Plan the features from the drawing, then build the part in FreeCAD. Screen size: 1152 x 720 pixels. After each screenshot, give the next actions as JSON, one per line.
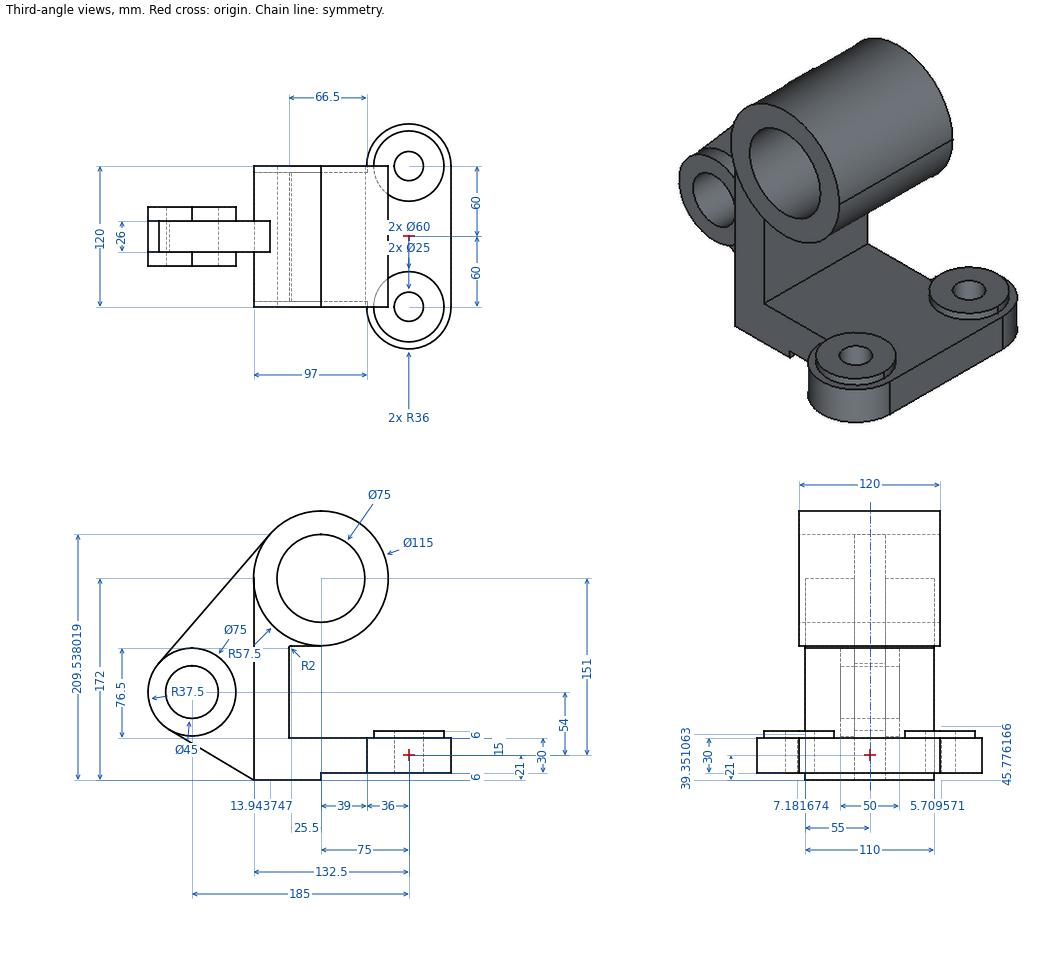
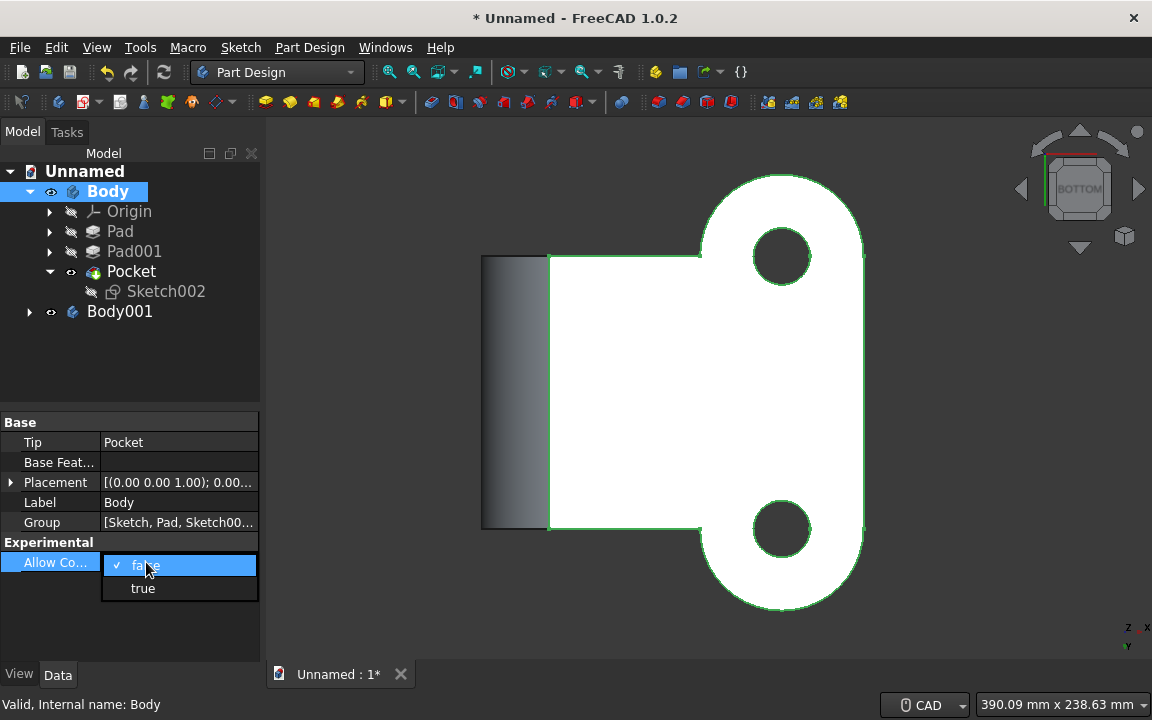
{"action": "left_click", "coordinate": [179, 588]}
{"action": "key", "text": "Return"}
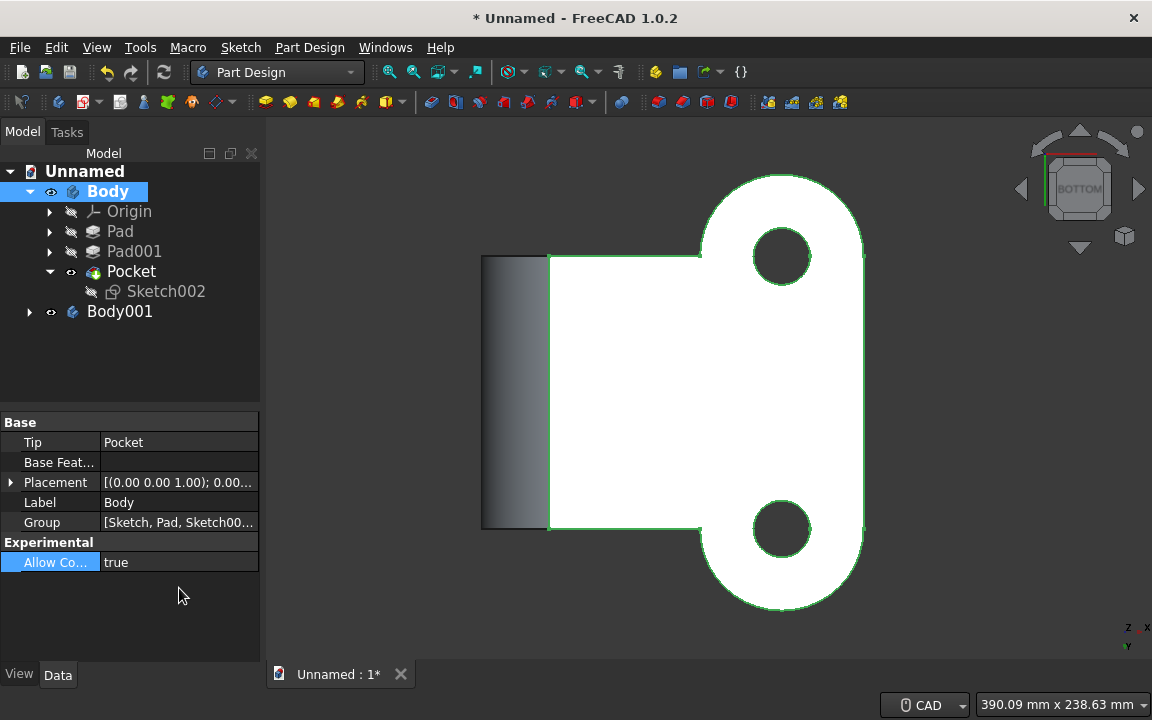
{"action": "left_click", "coordinate": [96, 312]}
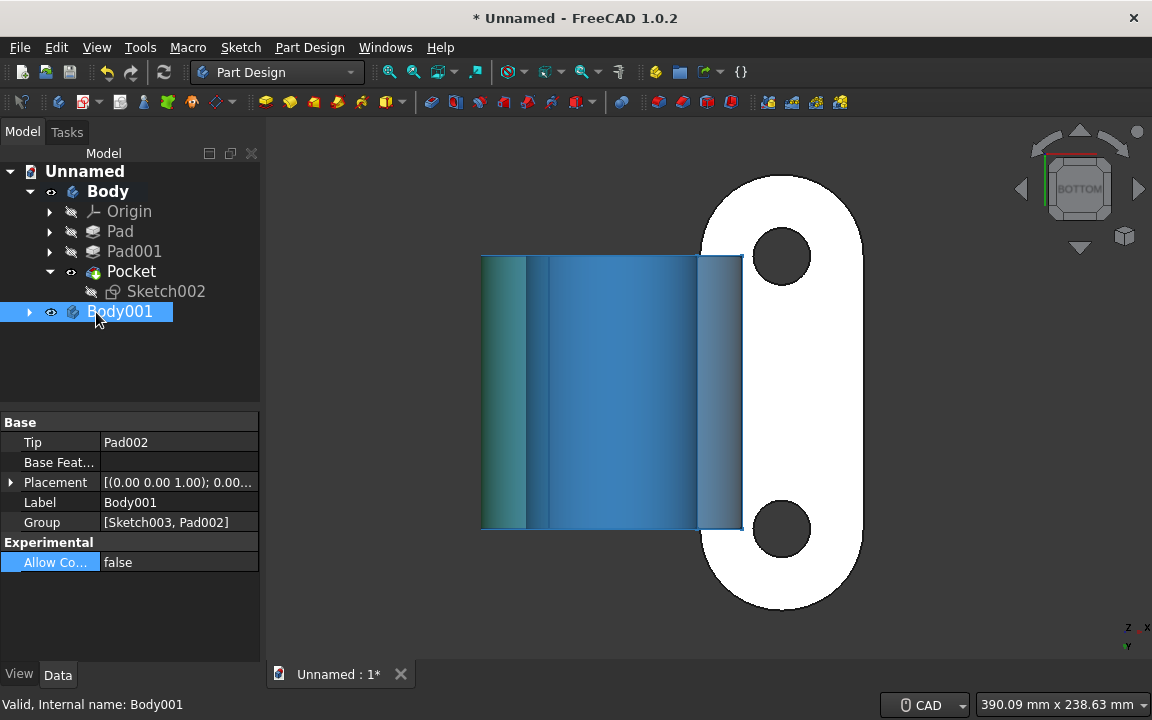
{"action": "left_click", "coordinate": [622, 102]}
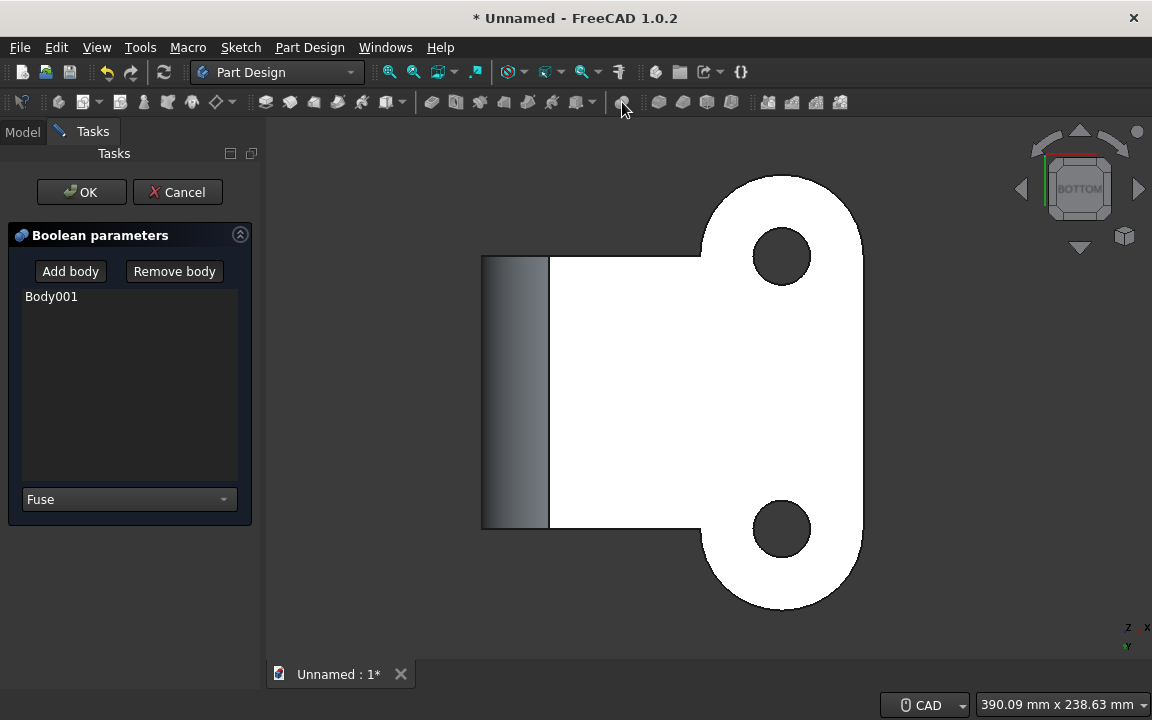
{"action": "left_click", "coordinate": [82, 192]}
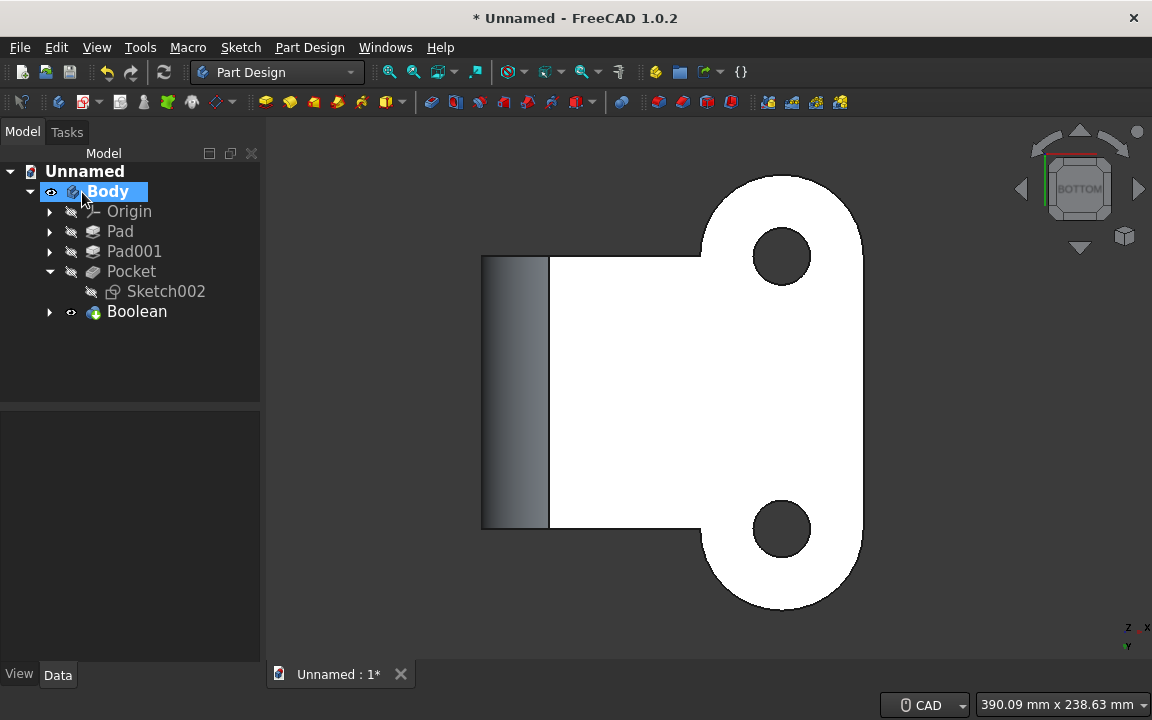
{"action": "left_click", "coordinate": [84, 102]}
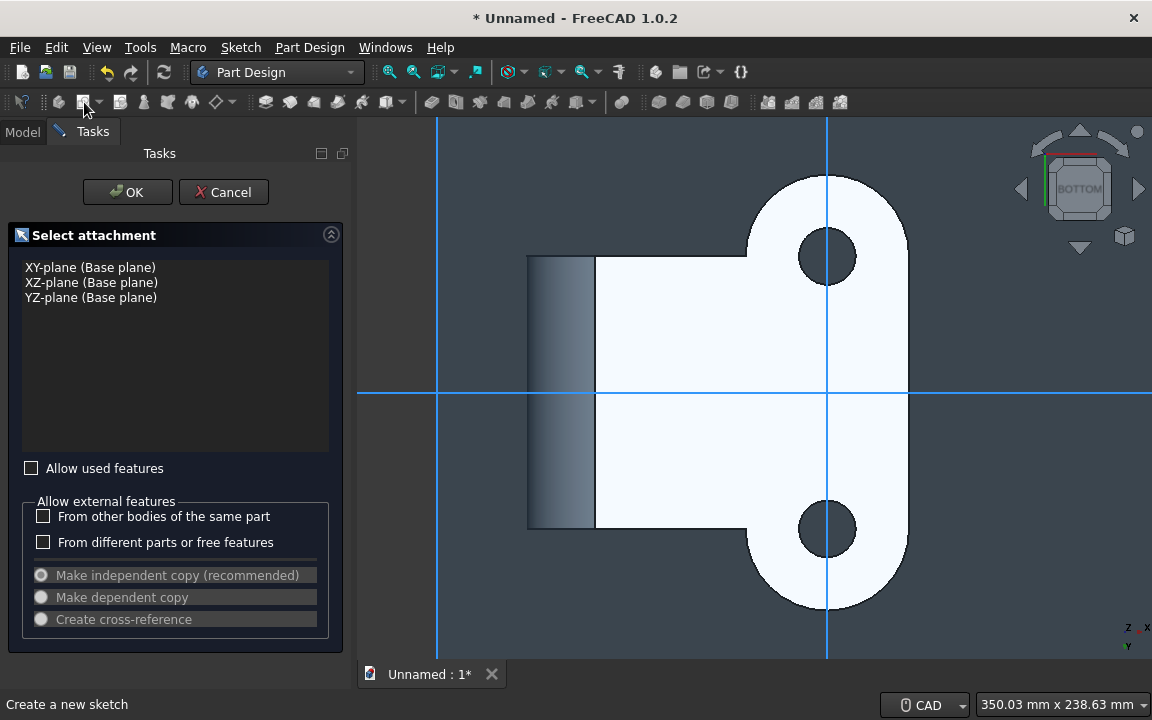
{"action": "left_click", "coordinate": [82, 282]}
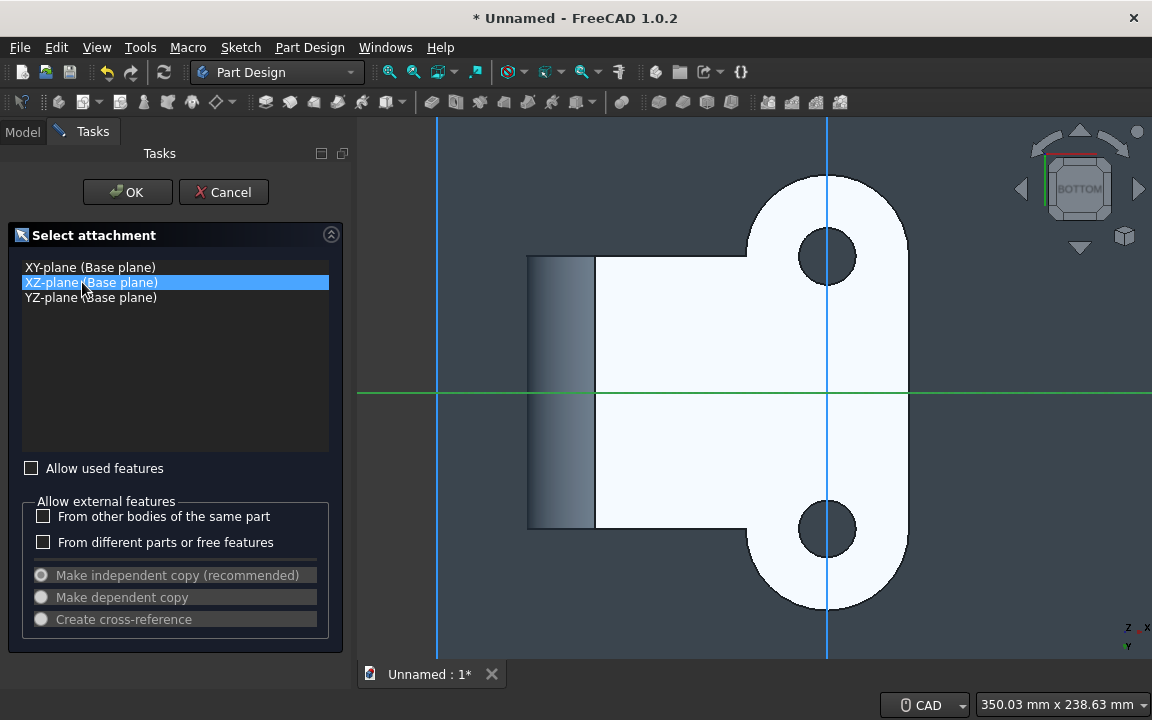
{"action": "left_click", "coordinate": [128, 192]}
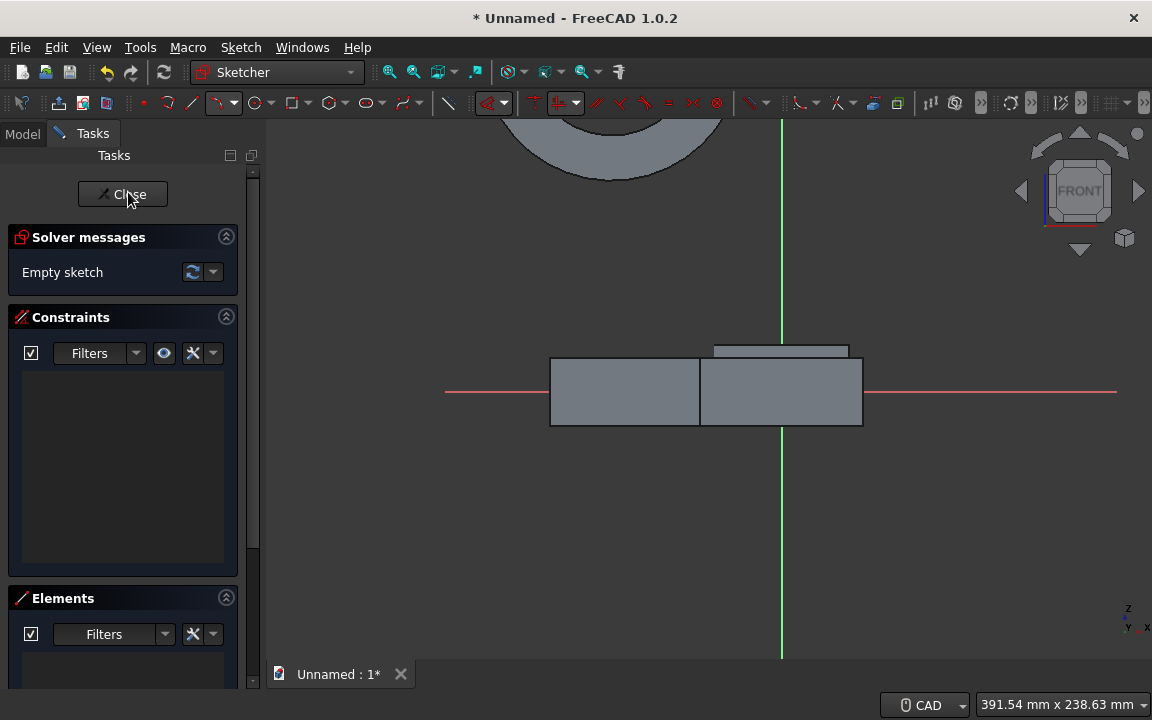
{"action": "key", "text": "q s"}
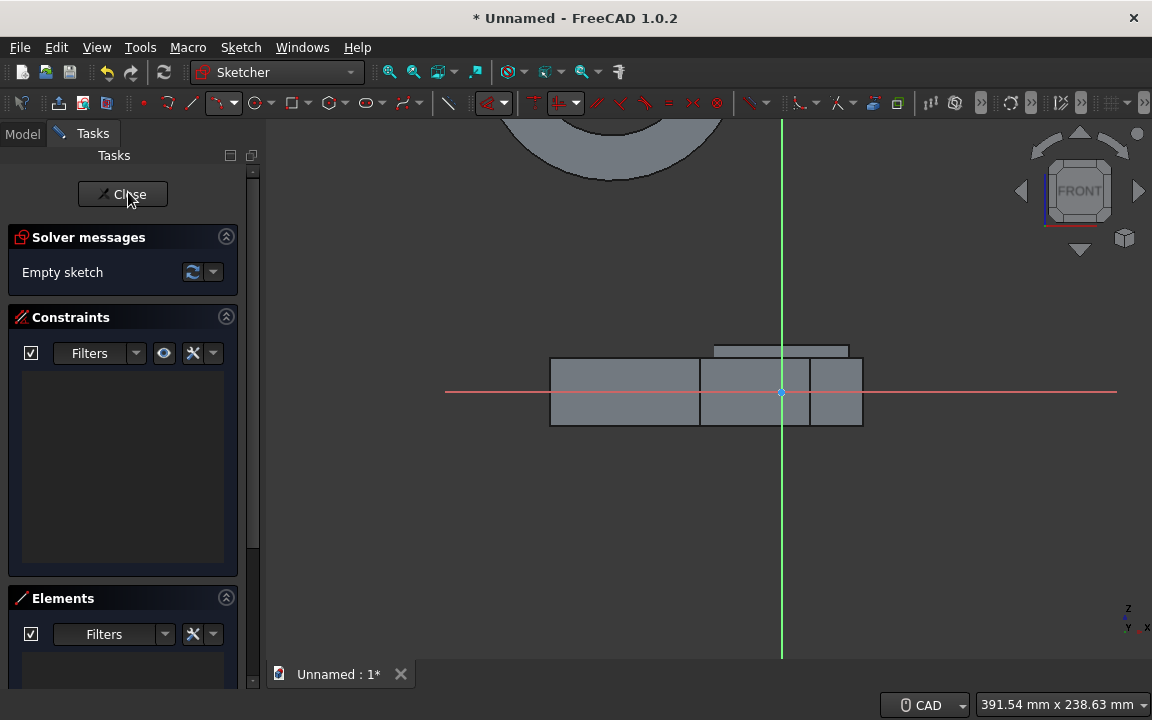
{"action": "scroll", "coordinate": [658, 631], "scroll_direction": "down", "scroll_amount": 2}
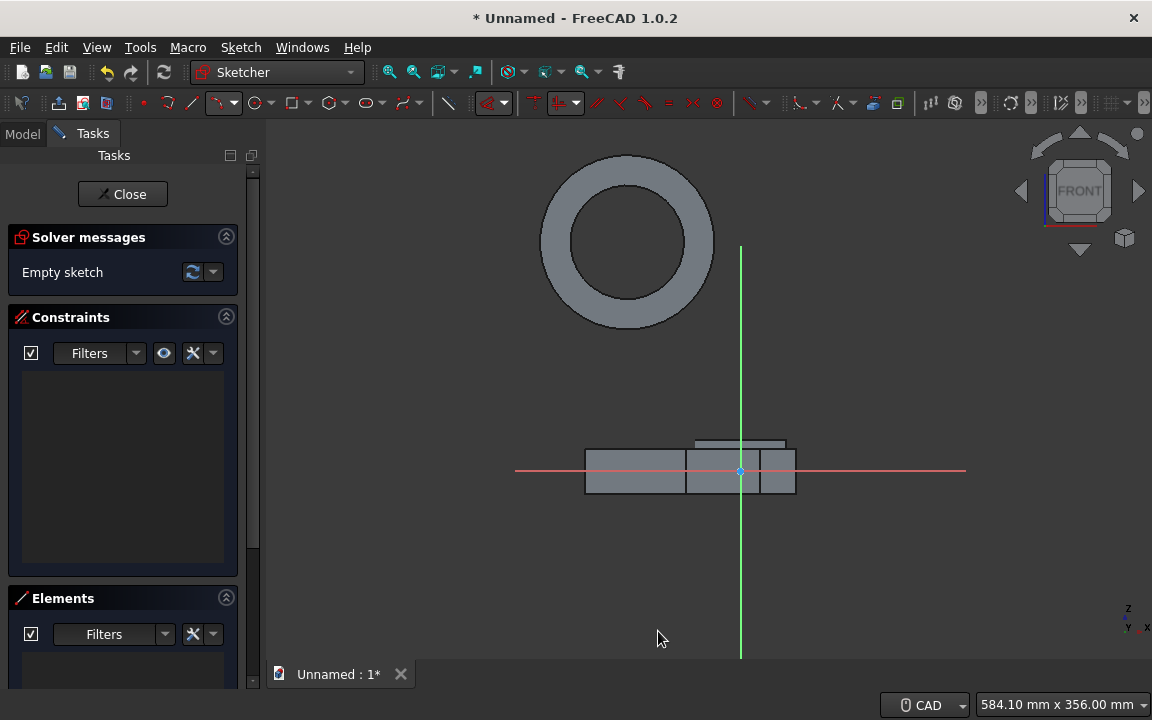
{"action": "left_click", "coordinate": [192, 104]}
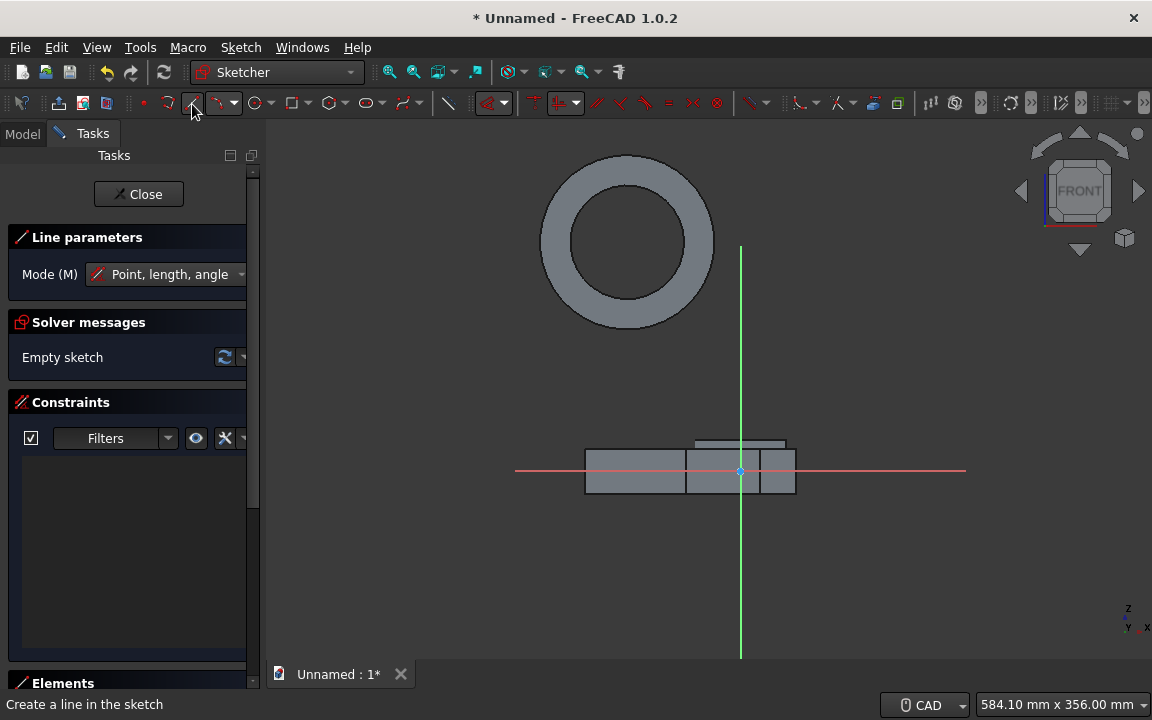
{"action": "left_click", "coordinate": [627, 330]}
{"action": "left_click", "coordinate": [589, 330]}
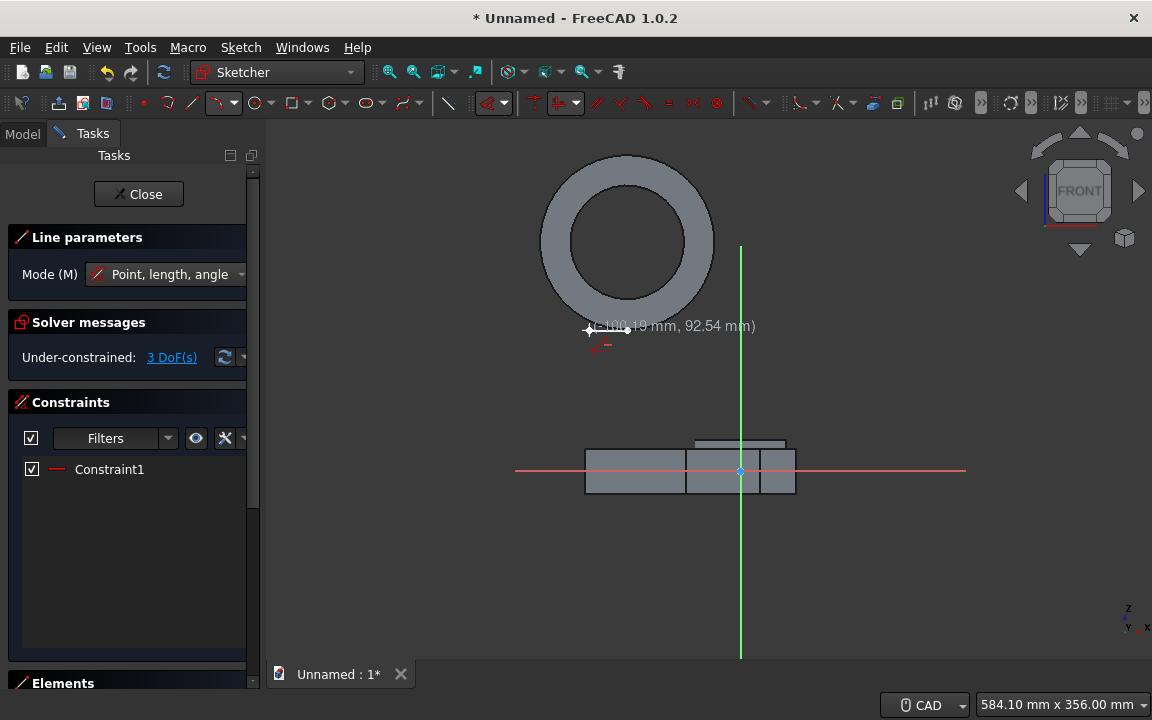
{"action": "left_click", "coordinate": [168, 104]}